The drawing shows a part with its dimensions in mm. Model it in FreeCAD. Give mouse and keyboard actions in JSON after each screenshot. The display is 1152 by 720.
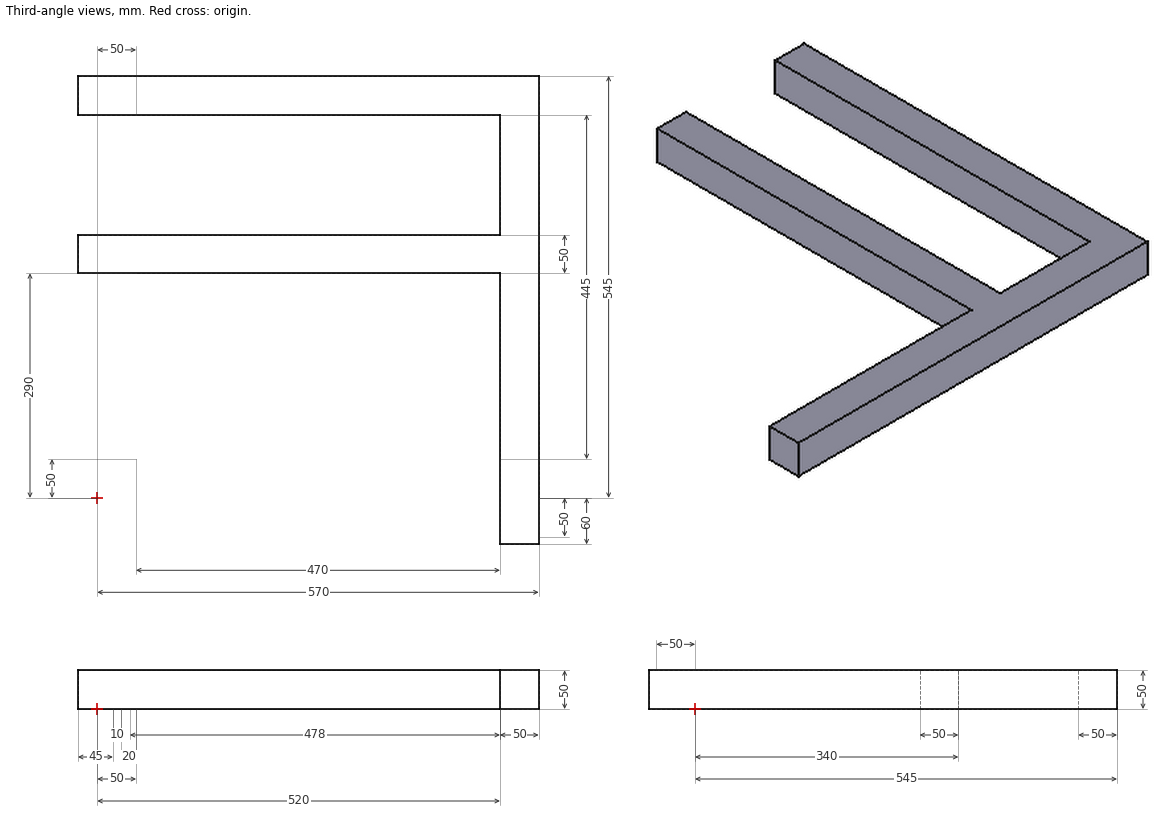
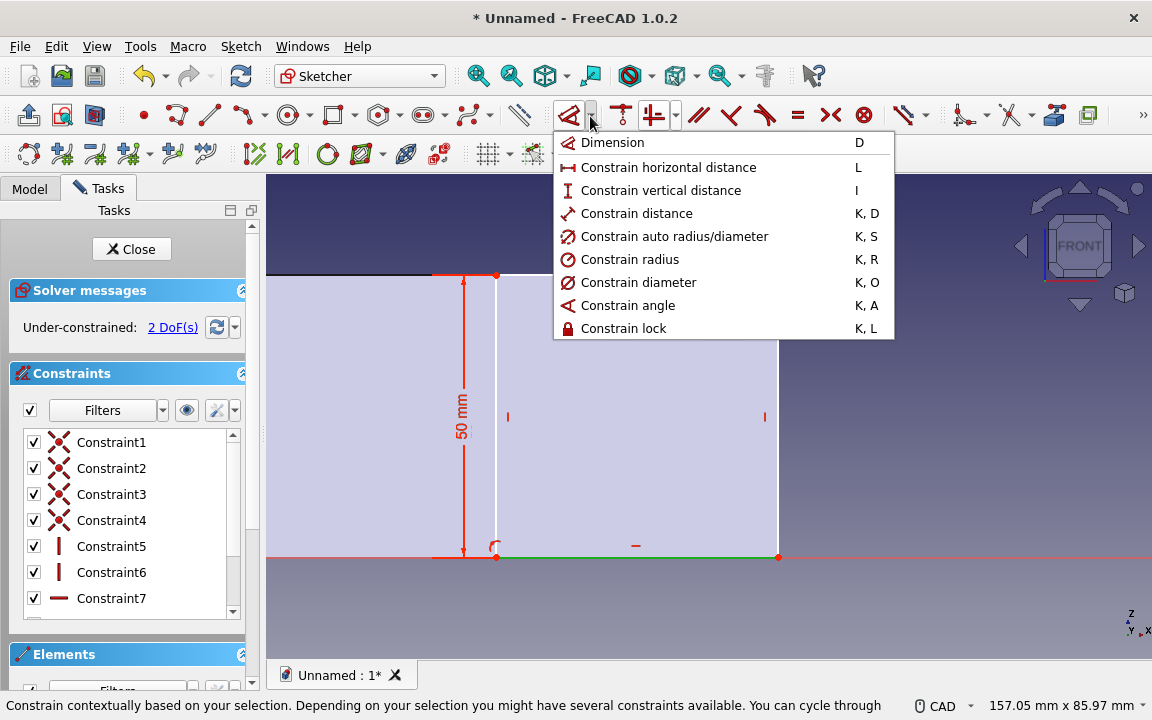
{"action": "left_click", "coordinate": [724, 168]}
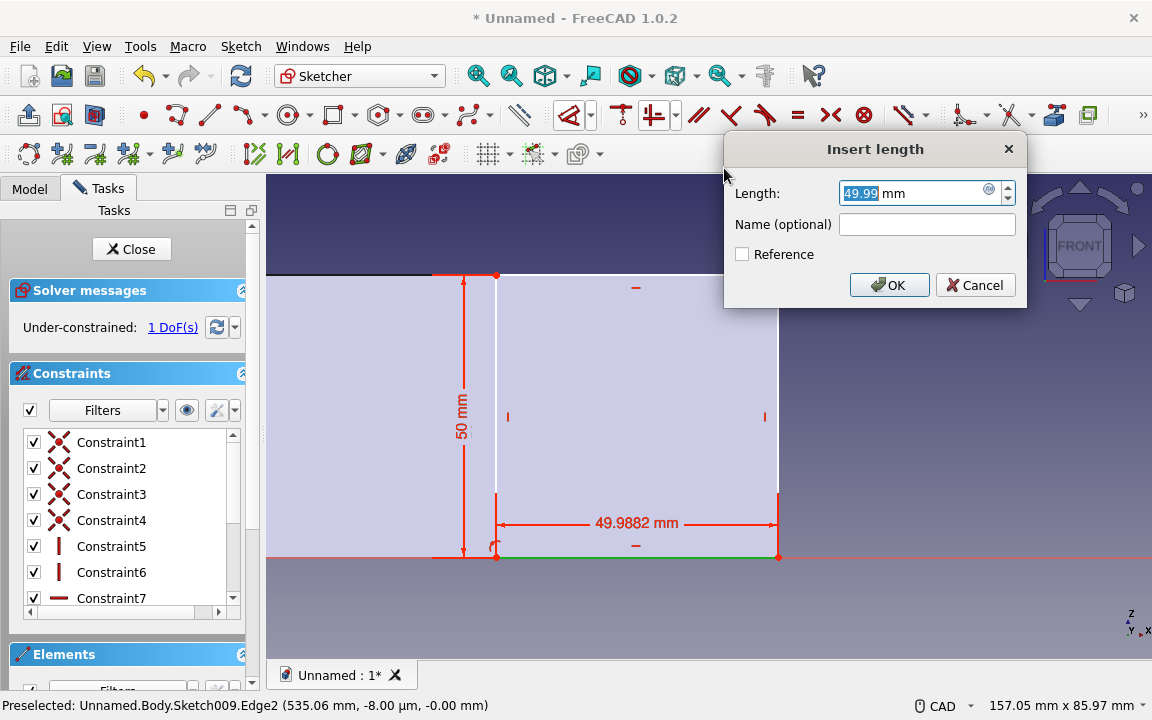
{"action": "type", "text": "50"}
{"action": "key", "text": "Return"}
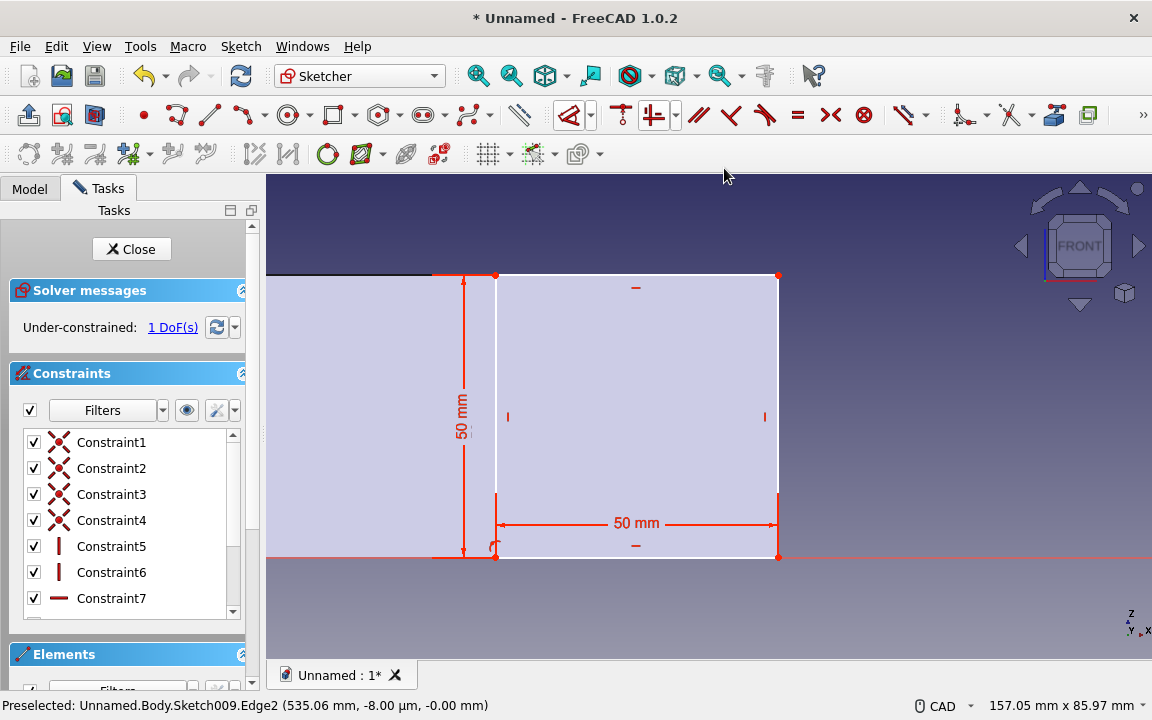
{"action": "left_click", "coordinate": [496, 275]}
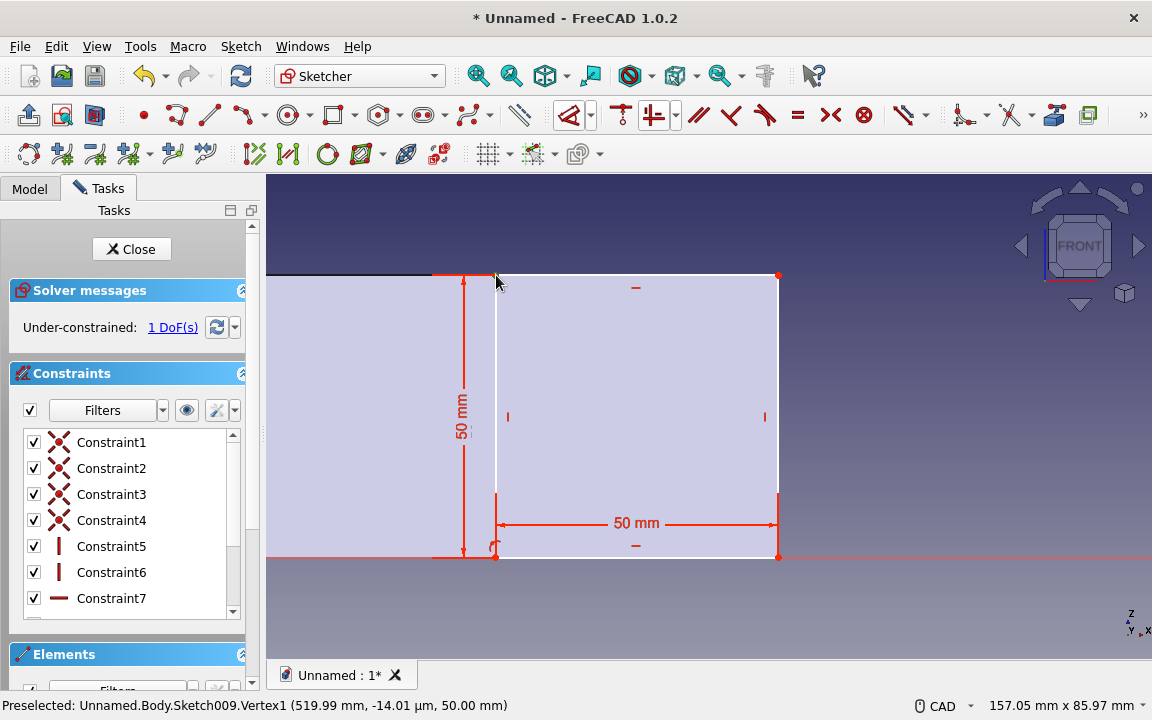
{"action": "key", "text": "l"}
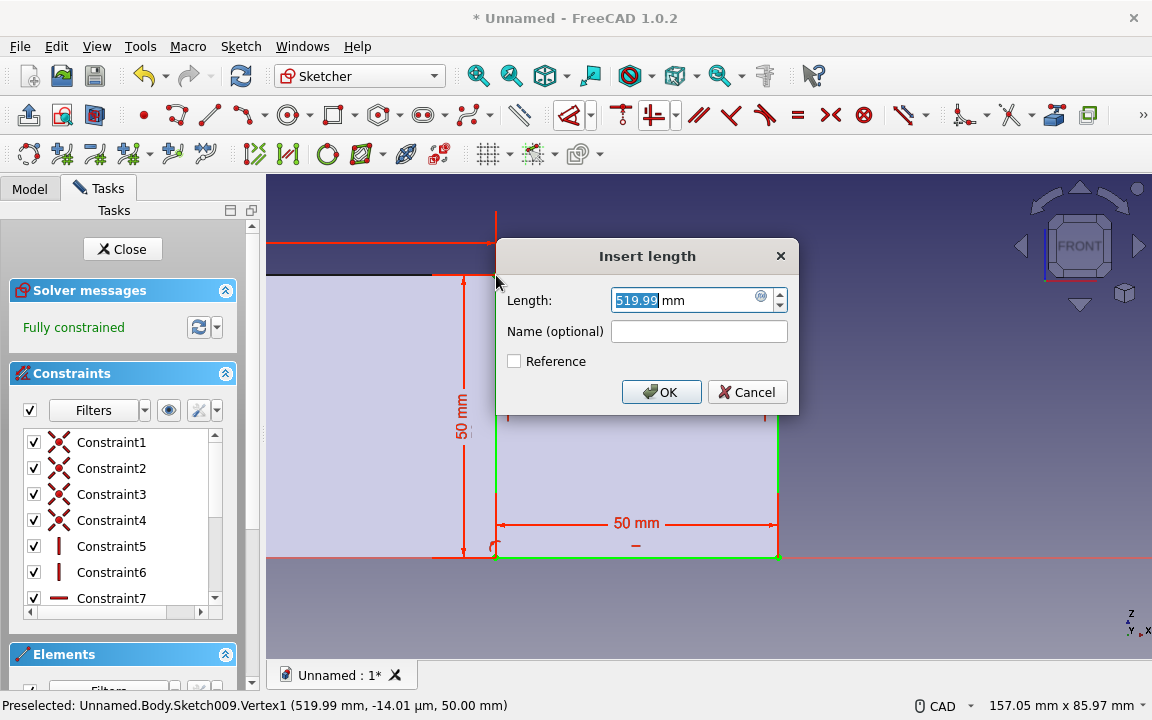
{"action": "type", "text": "520"}
{"action": "key", "text": "Return"}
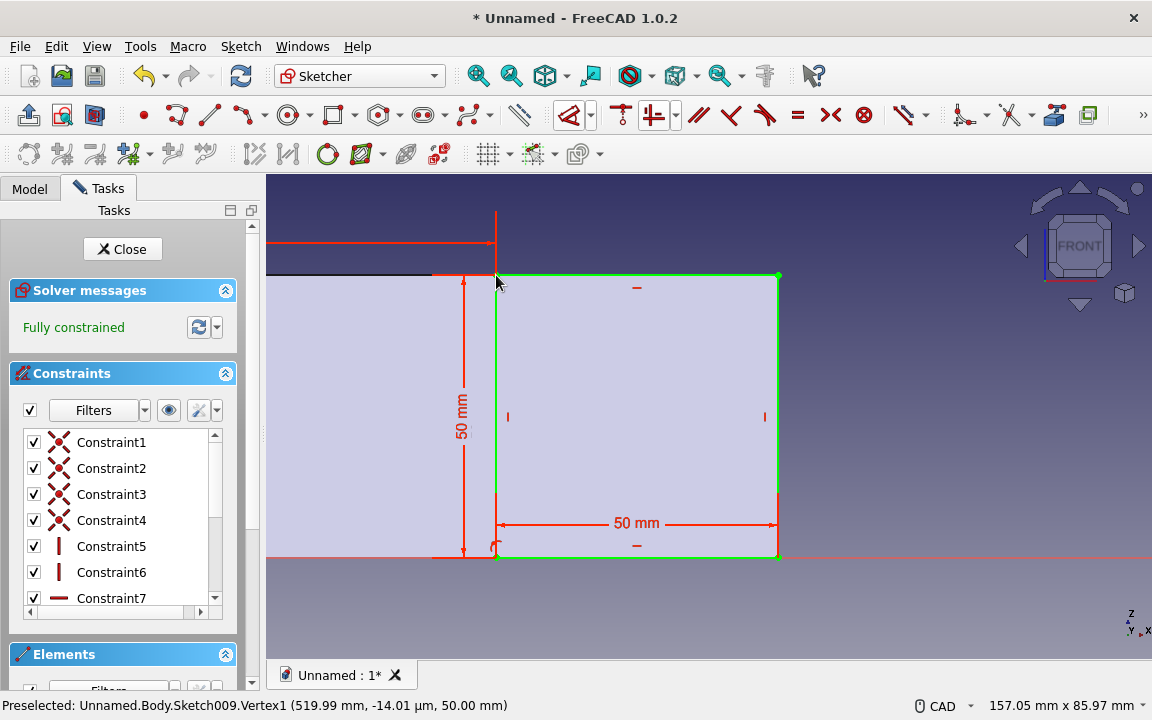
{"action": "left_click", "coordinate": [123, 249]}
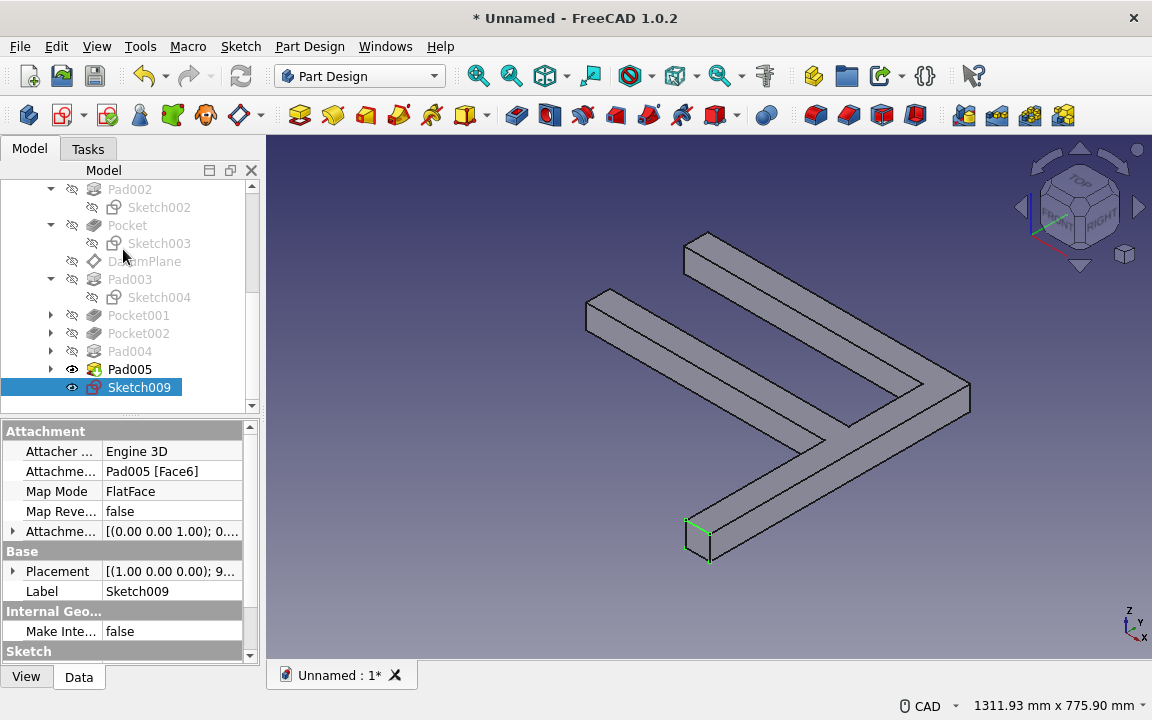
{"action": "left_click", "coordinate": [300, 116]}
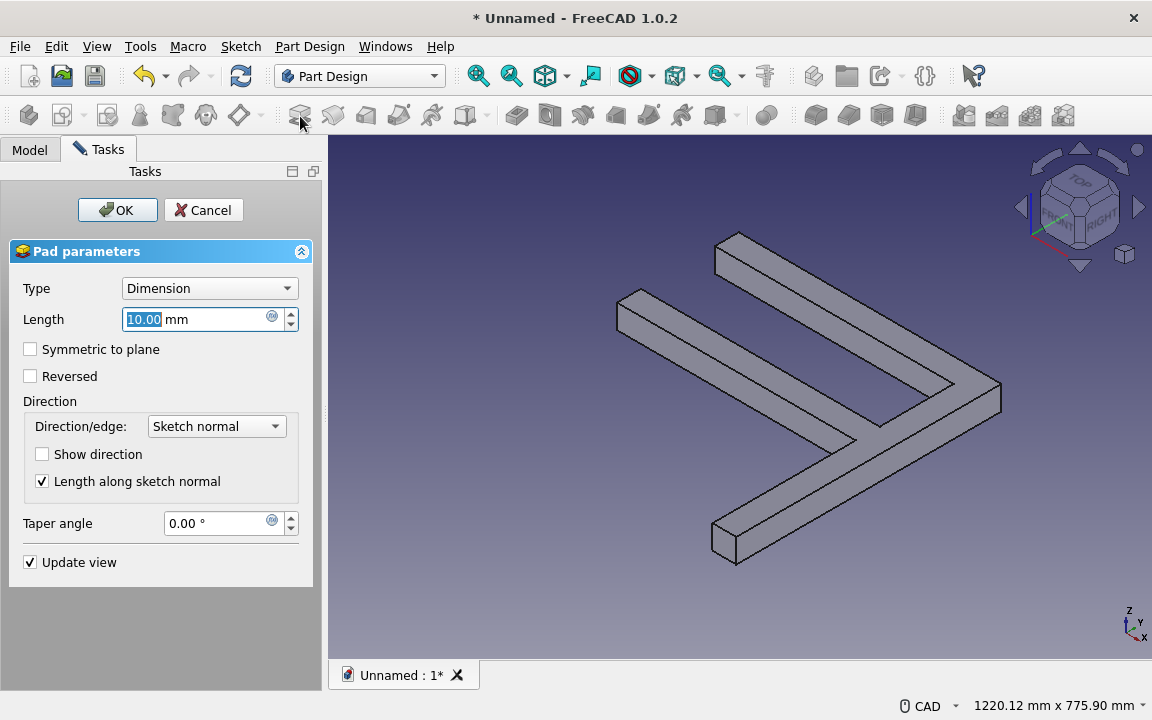
{"action": "type", "text": "60"}
{"action": "key", "text": "Tab"}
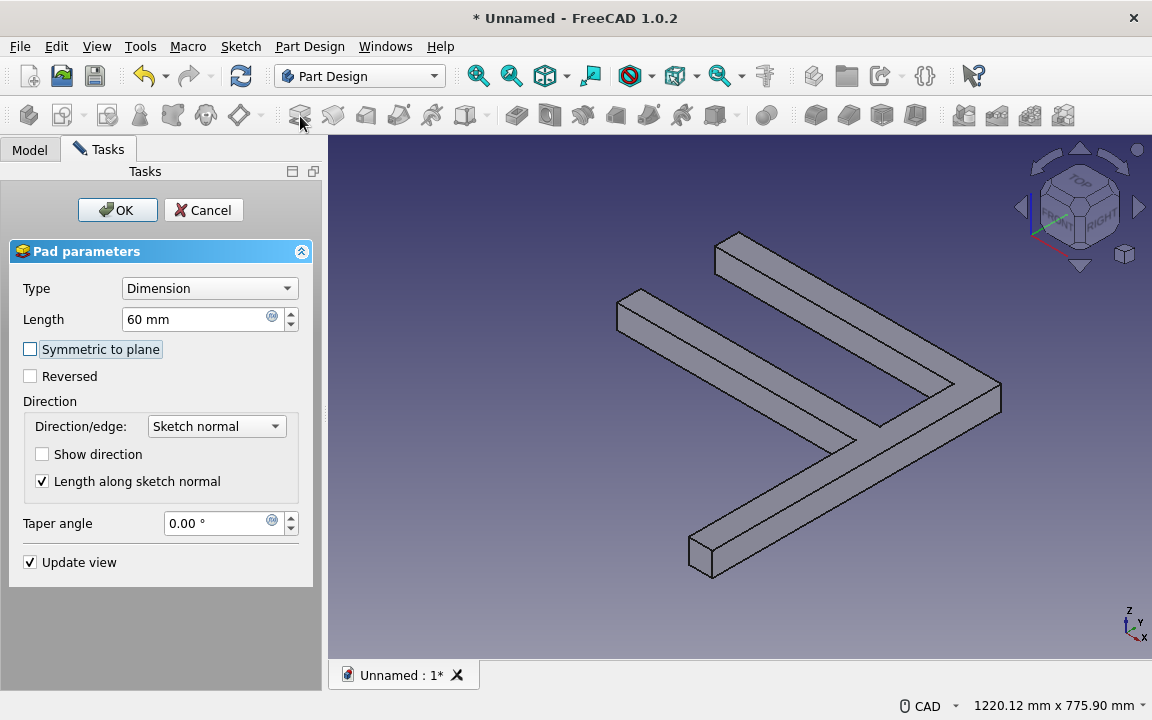
{"action": "left_click", "coordinate": [118, 210]}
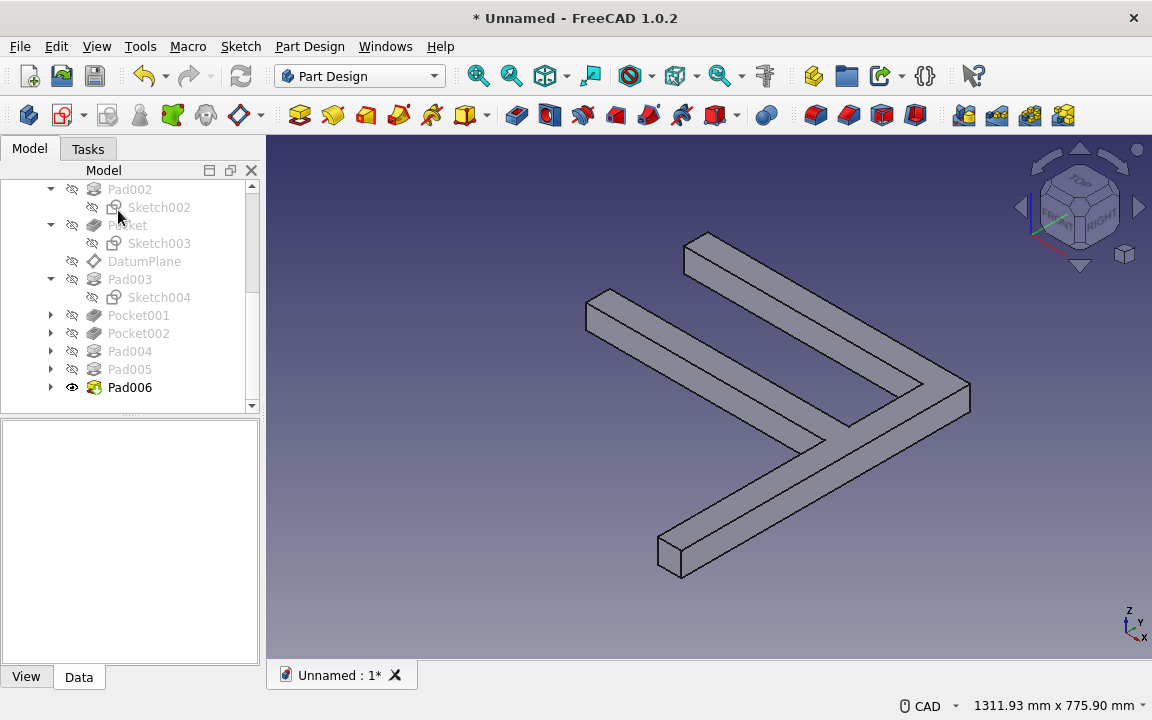
{"action": "key", "text": "6"}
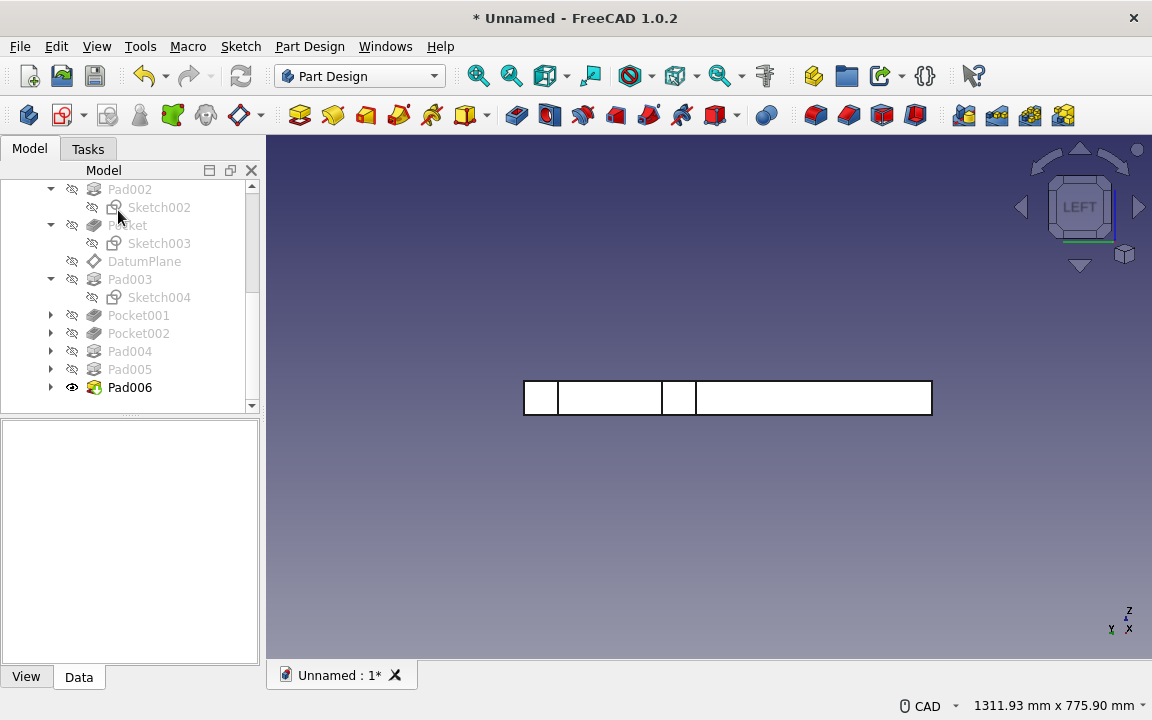
{"action": "left_click", "coordinate": [541, 397]}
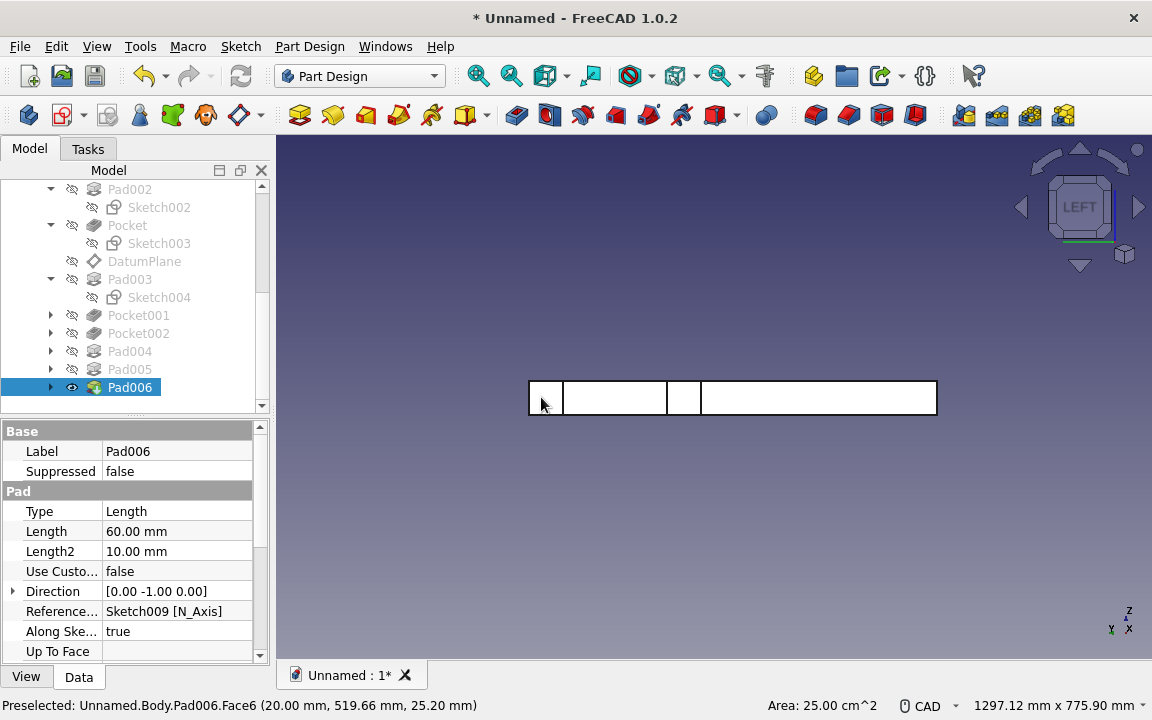
{"action": "left_click", "coordinate": [62, 116]}